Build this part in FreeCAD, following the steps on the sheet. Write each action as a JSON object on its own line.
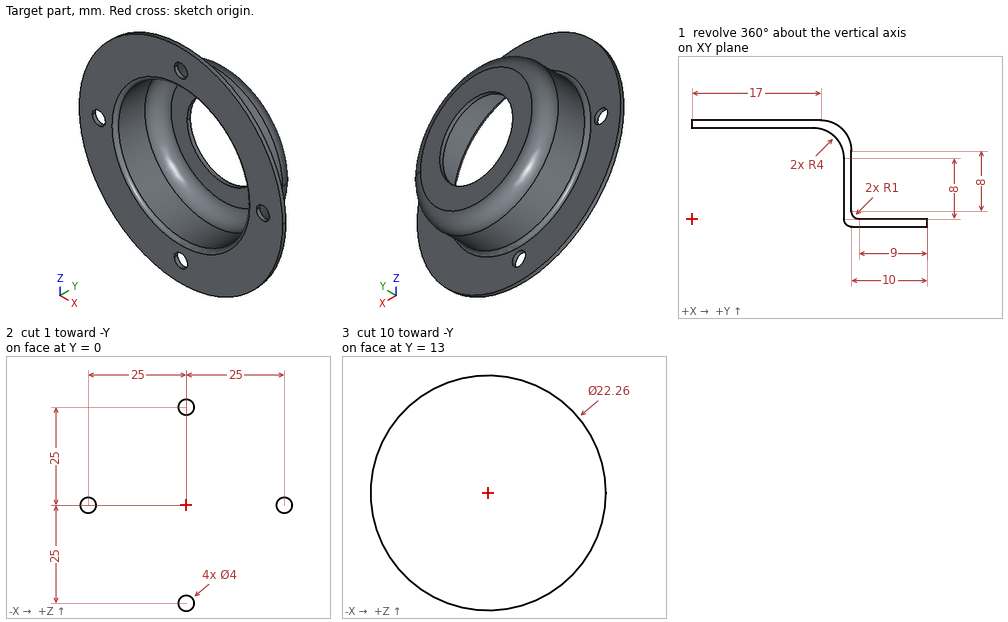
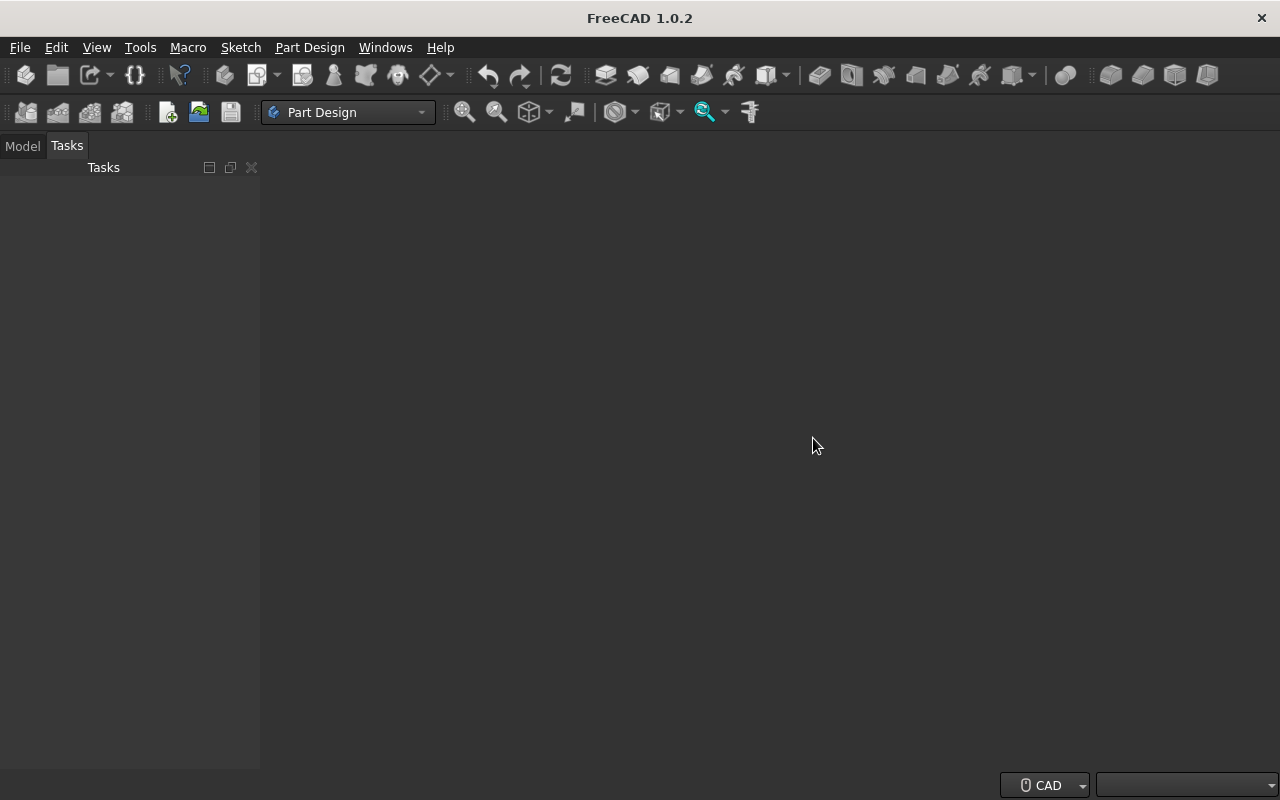
{"action": "left_click", "coordinate": [168, 112]}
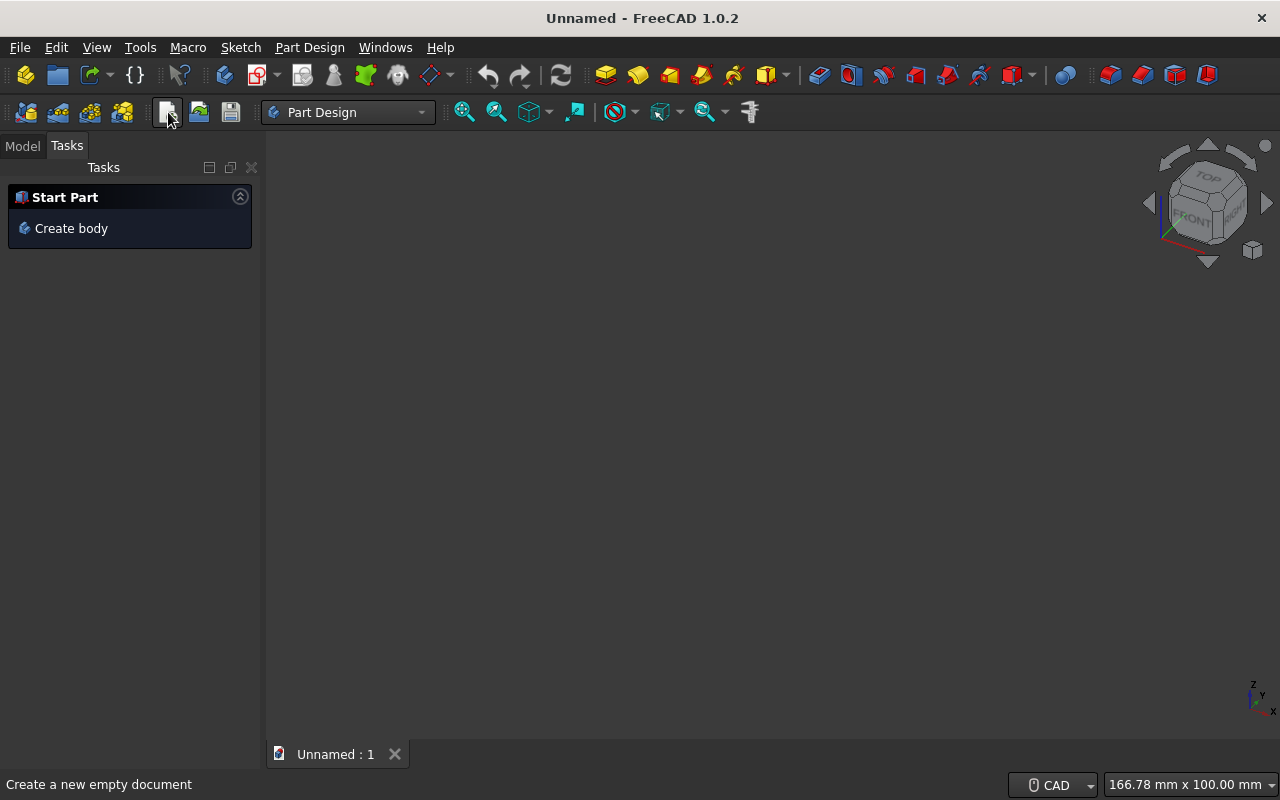
{"action": "left_click", "coordinate": [258, 76]}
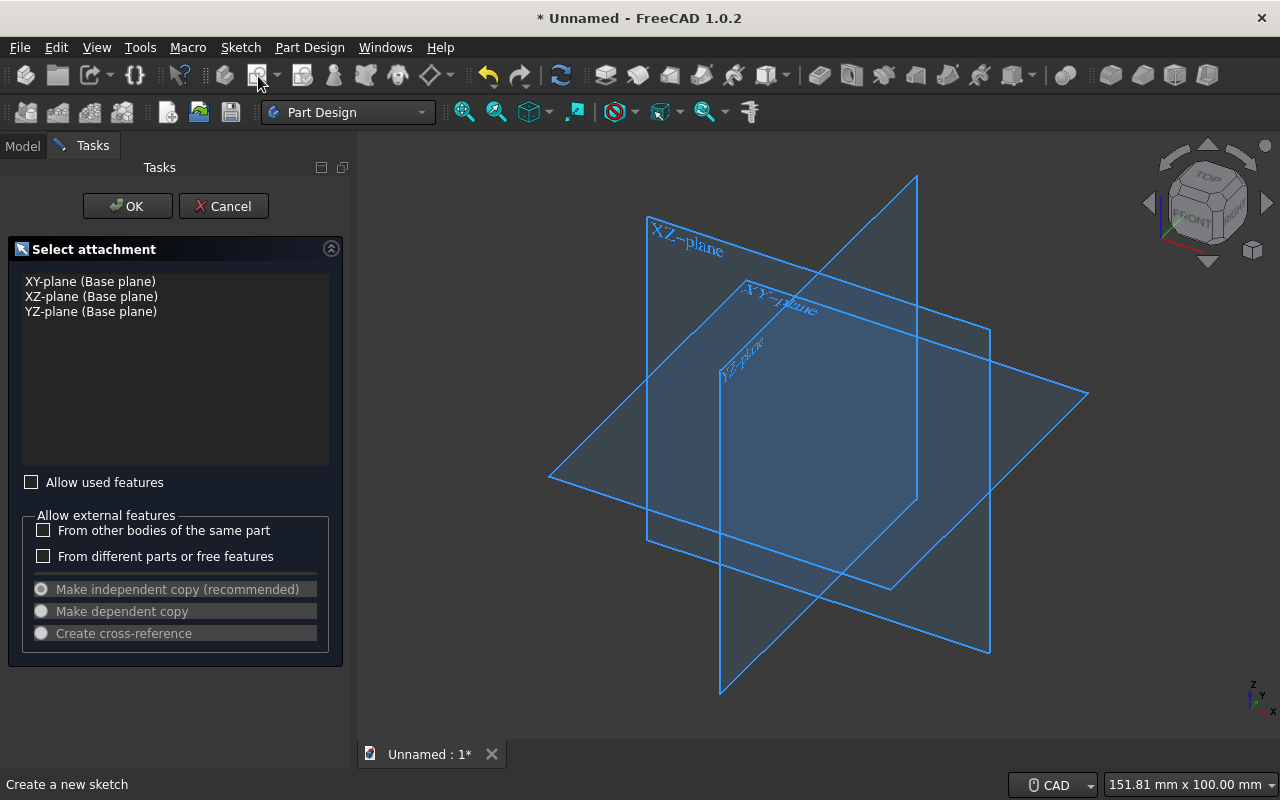
{"action": "left_click", "coordinate": [82, 282]}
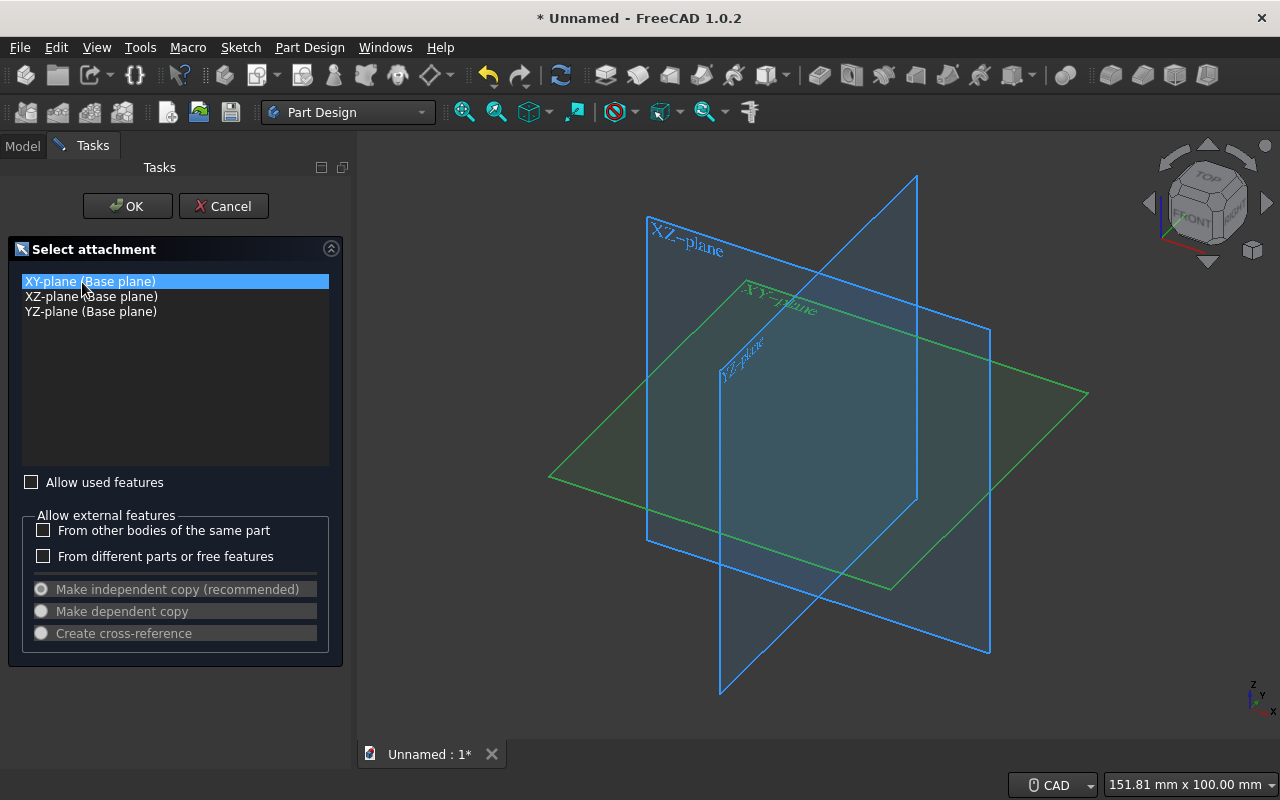
{"action": "left_click", "coordinate": [128, 206]}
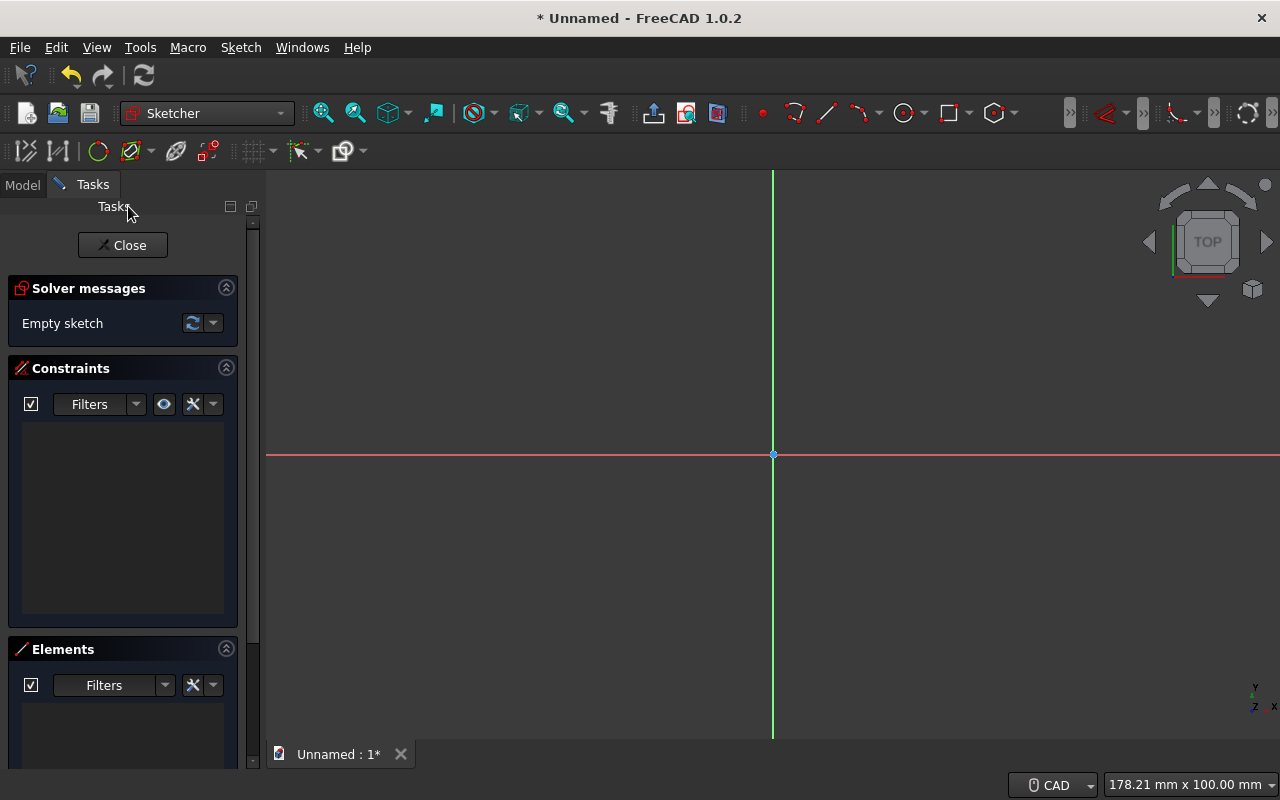
{"action": "scroll", "coordinate": [929, 406], "scroll_direction": "up", "scroll_amount": 6}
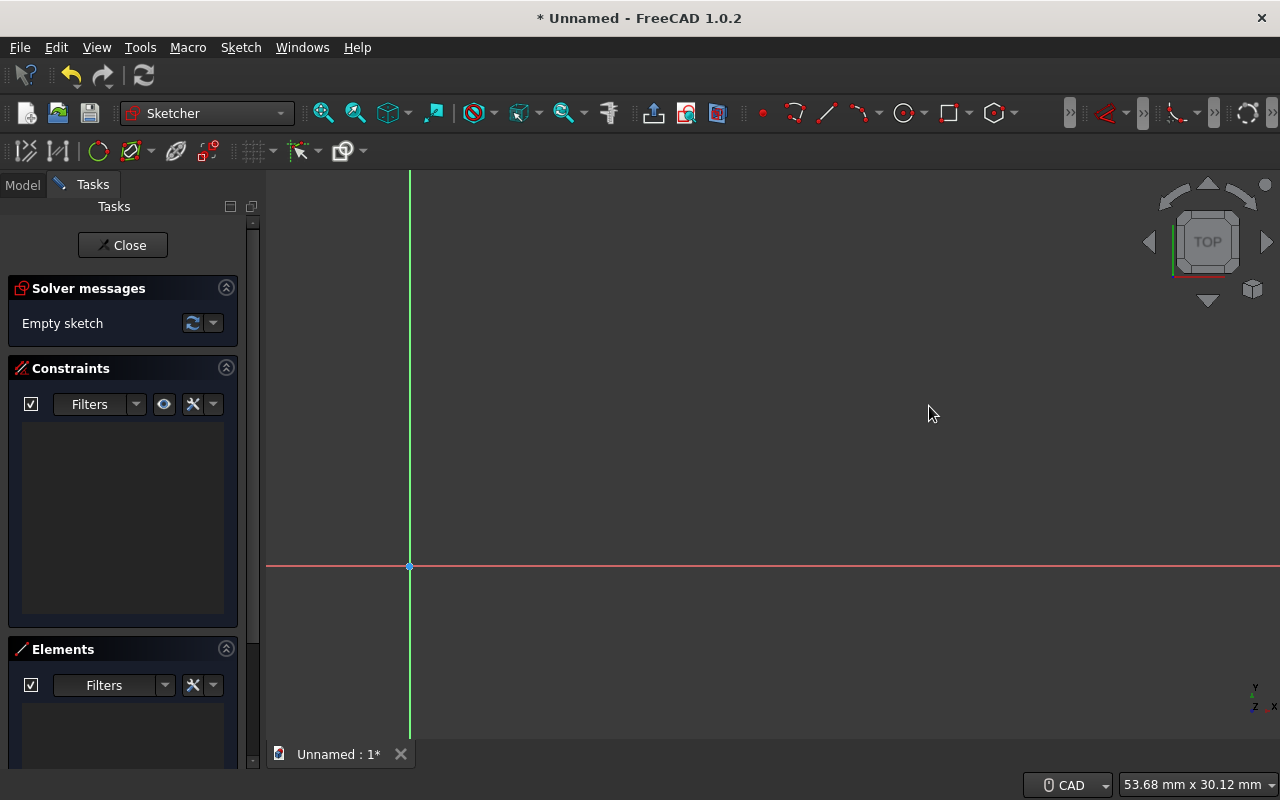
{"action": "key", "text": "g l"}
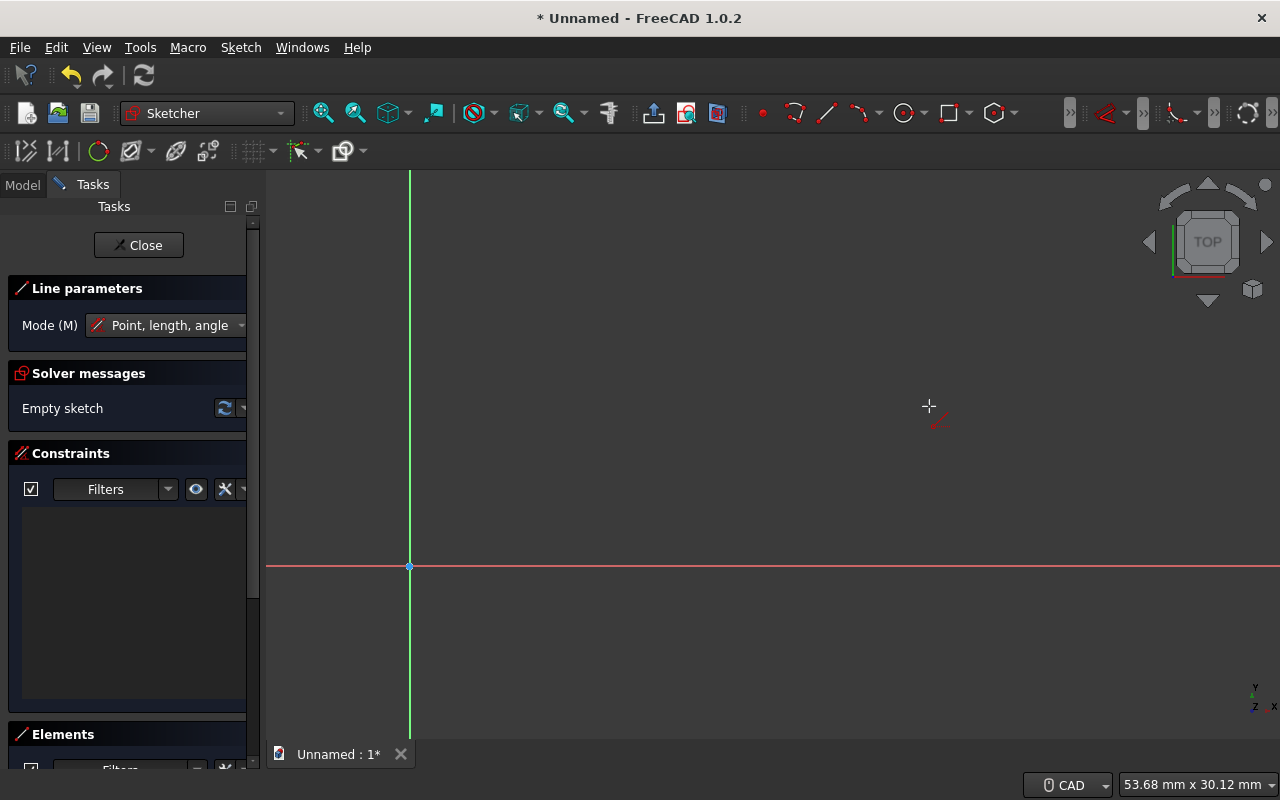
{"action": "left_click", "coordinate": [787, 415]}
{"action": "left_click", "coordinate": [787, 566]}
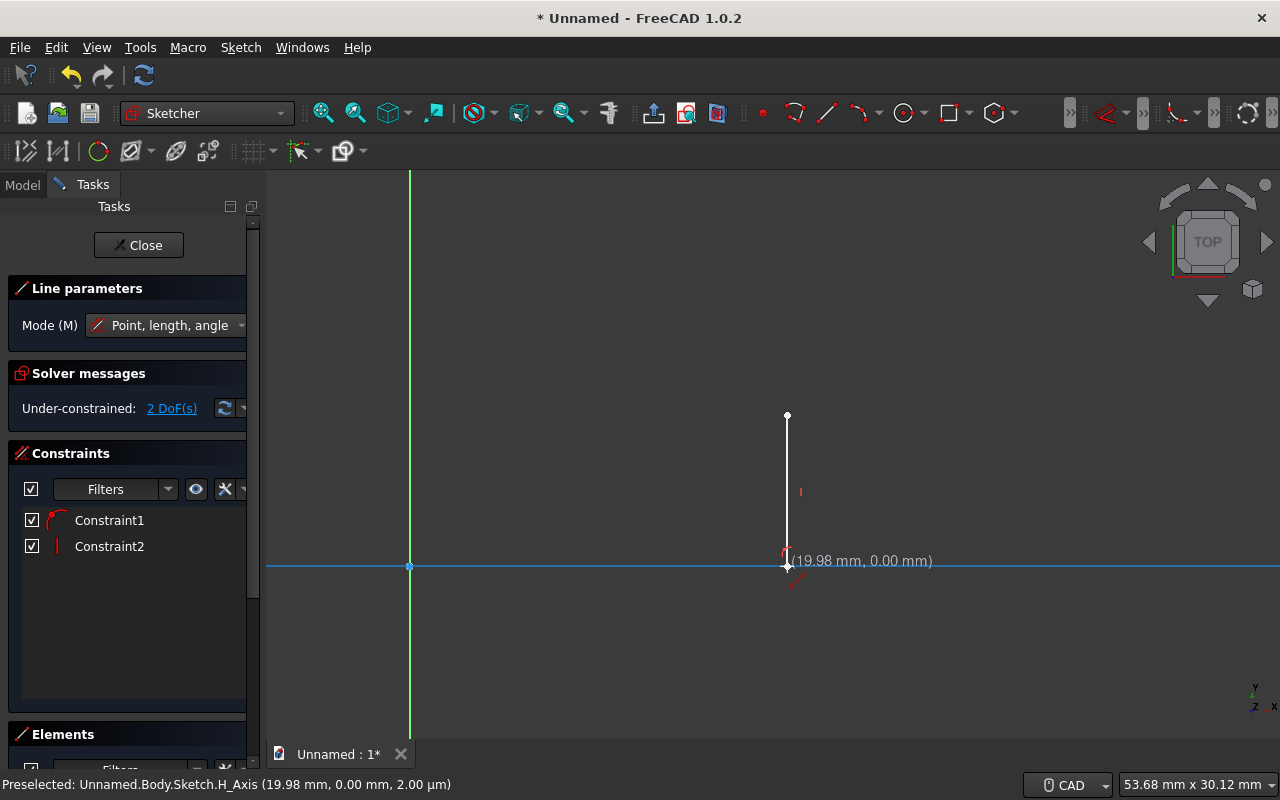
{"action": "left_click", "coordinate": [796, 114]}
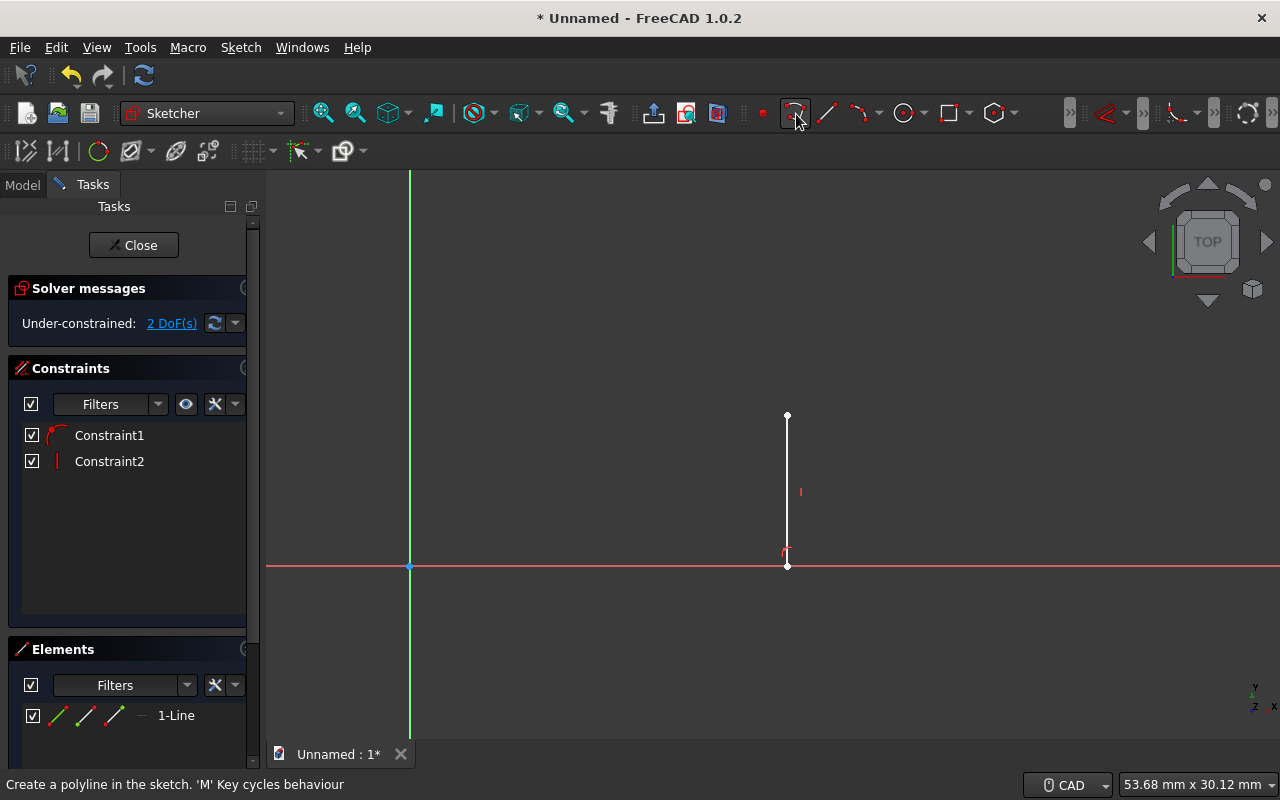
{"action": "left_click", "coordinate": [806, 585]}
{"action": "left_click", "coordinate": [995, 585]}
{"action": "left_click", "coordinate": [995, 566]}
{"action": "left_click", "coordinate": [825, 557]}
{"action": "right_click", "coordinate": [825, 557]}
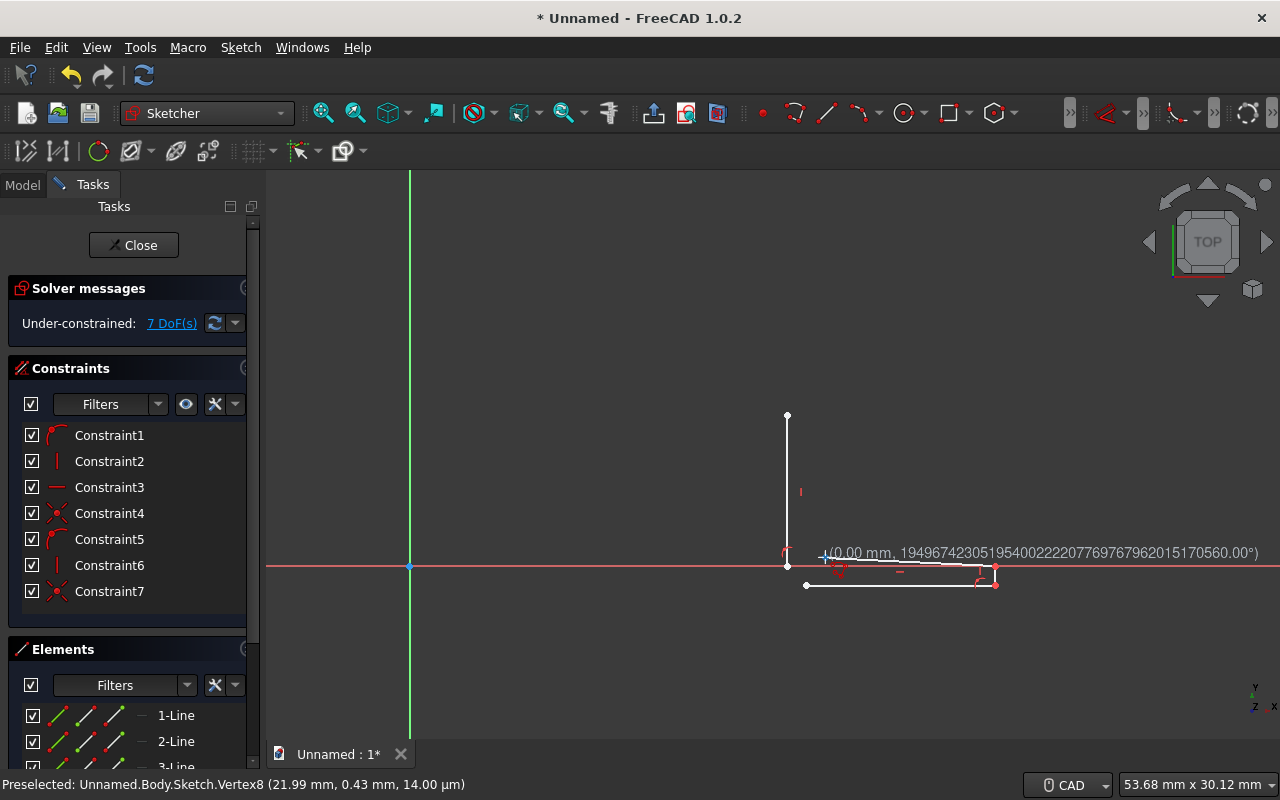
{"action": "left_click", "coordinate": [828, 114]}